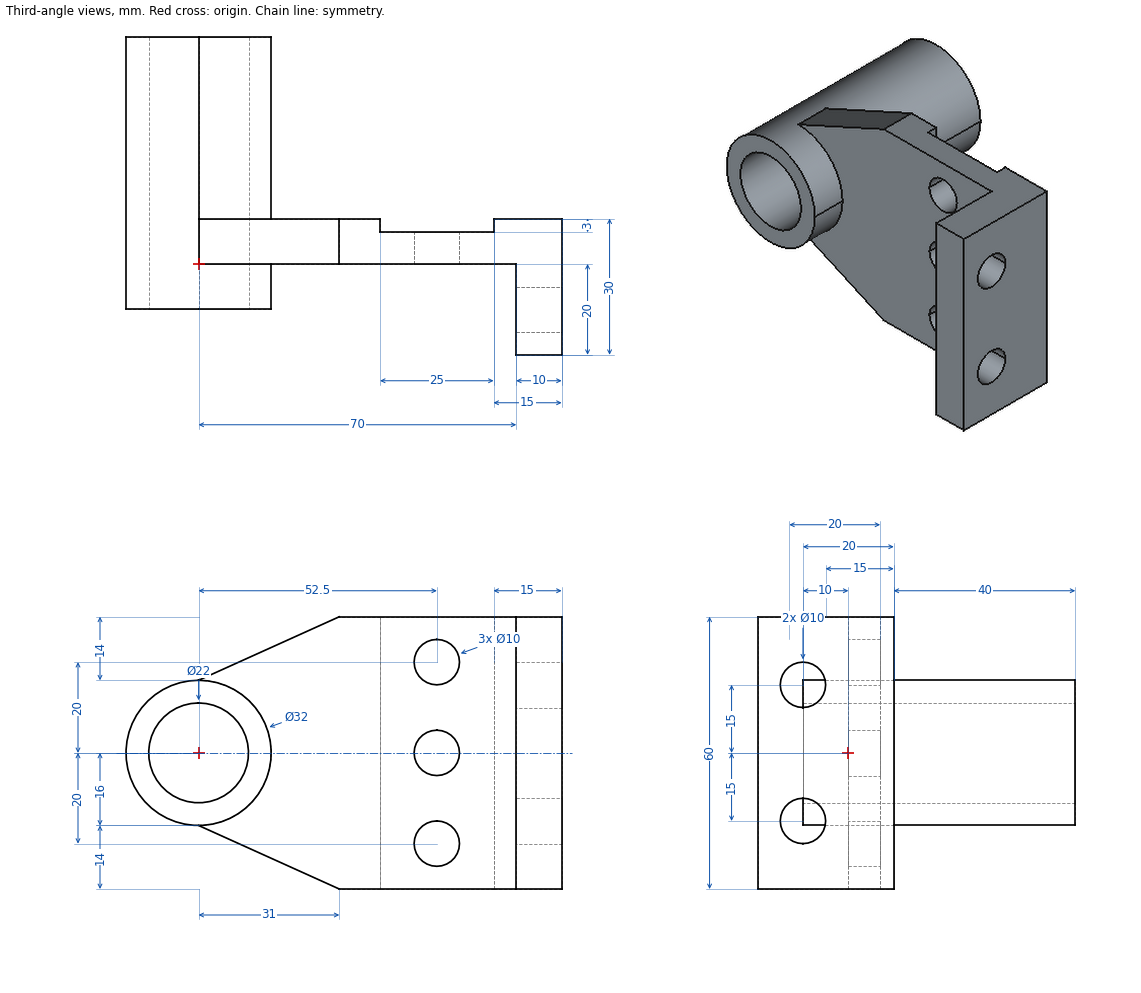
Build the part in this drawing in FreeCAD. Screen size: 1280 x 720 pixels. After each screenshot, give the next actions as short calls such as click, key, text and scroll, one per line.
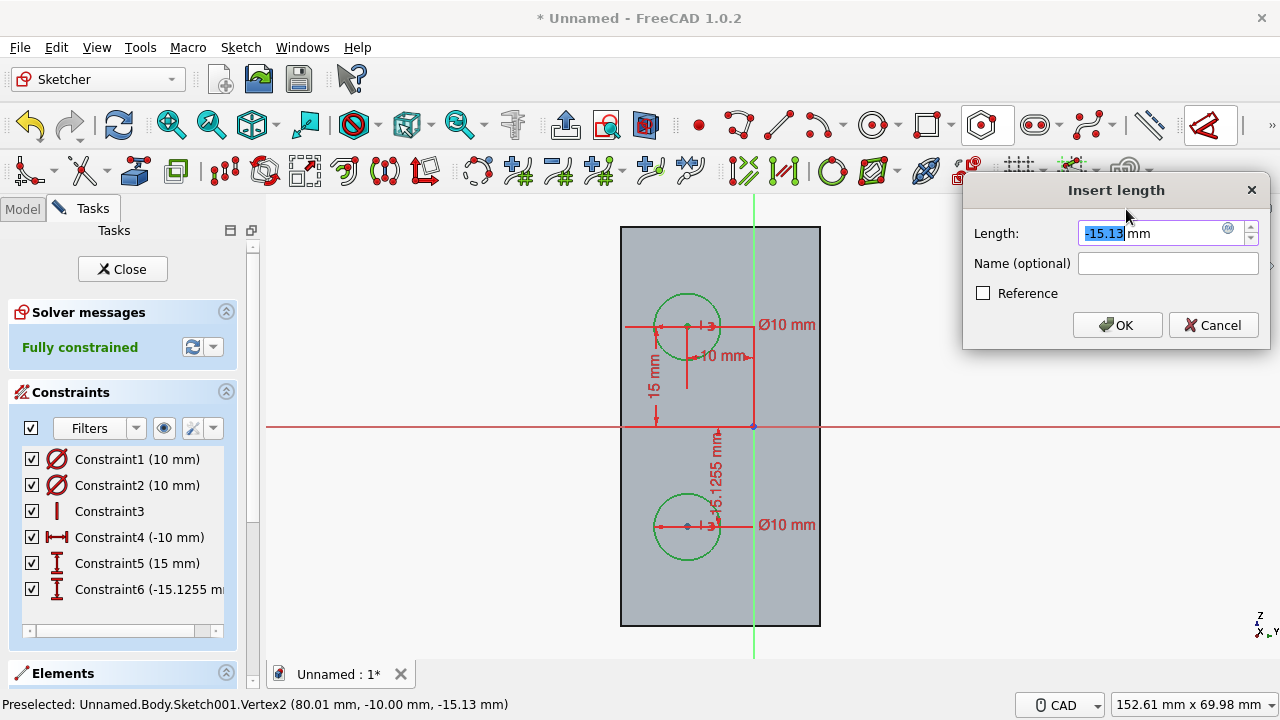
text(-15)
key(Return)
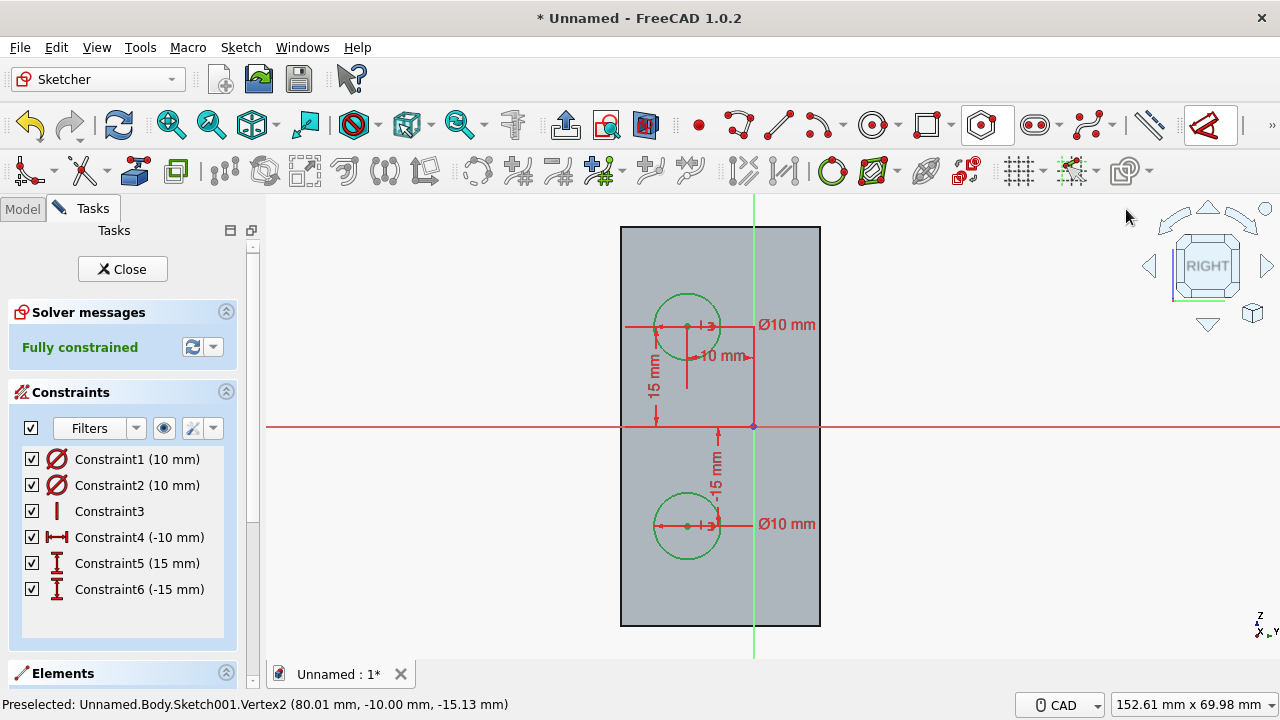
click(123, 269)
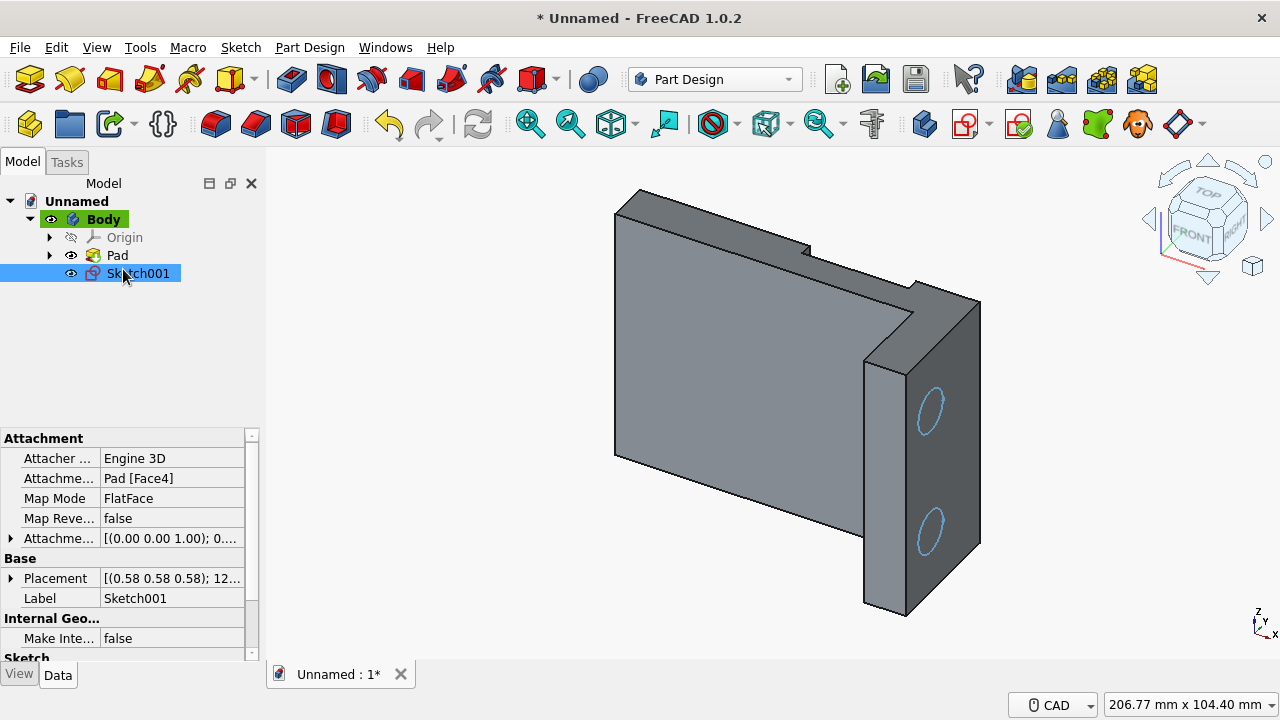
click(292, 80)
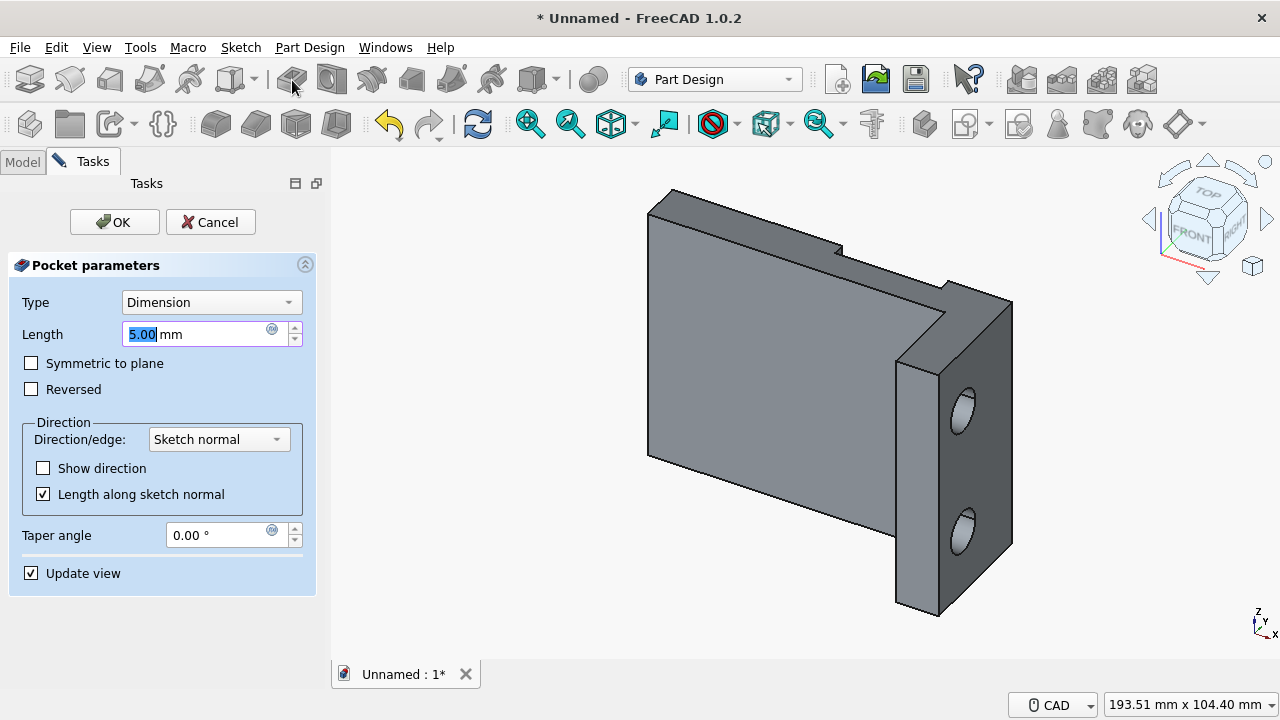
text(15)
key(Tab)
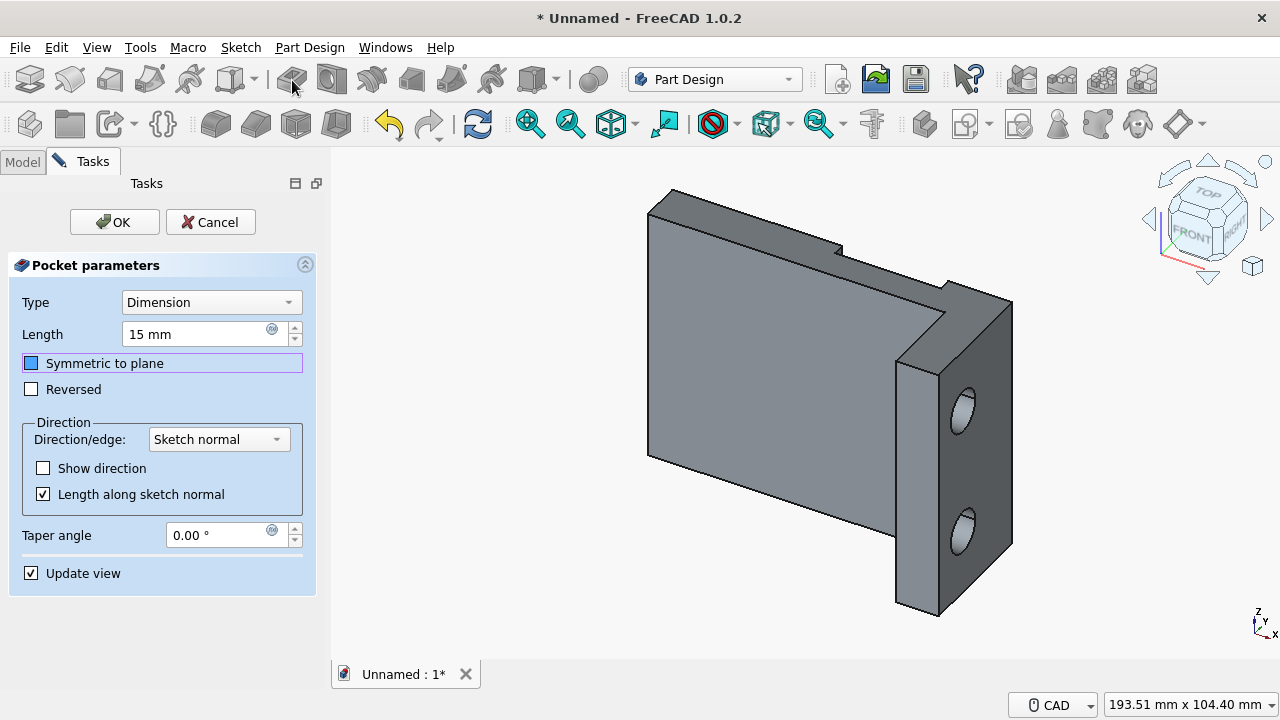
click(115, 222)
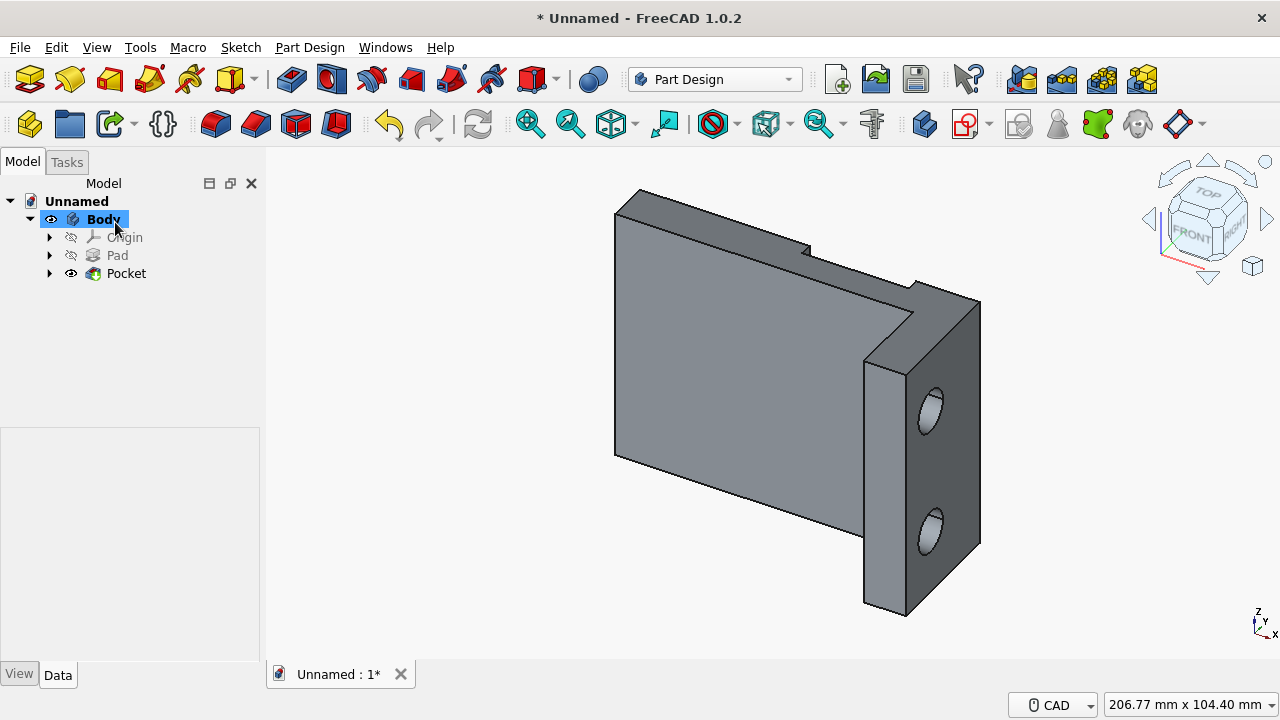
key(4)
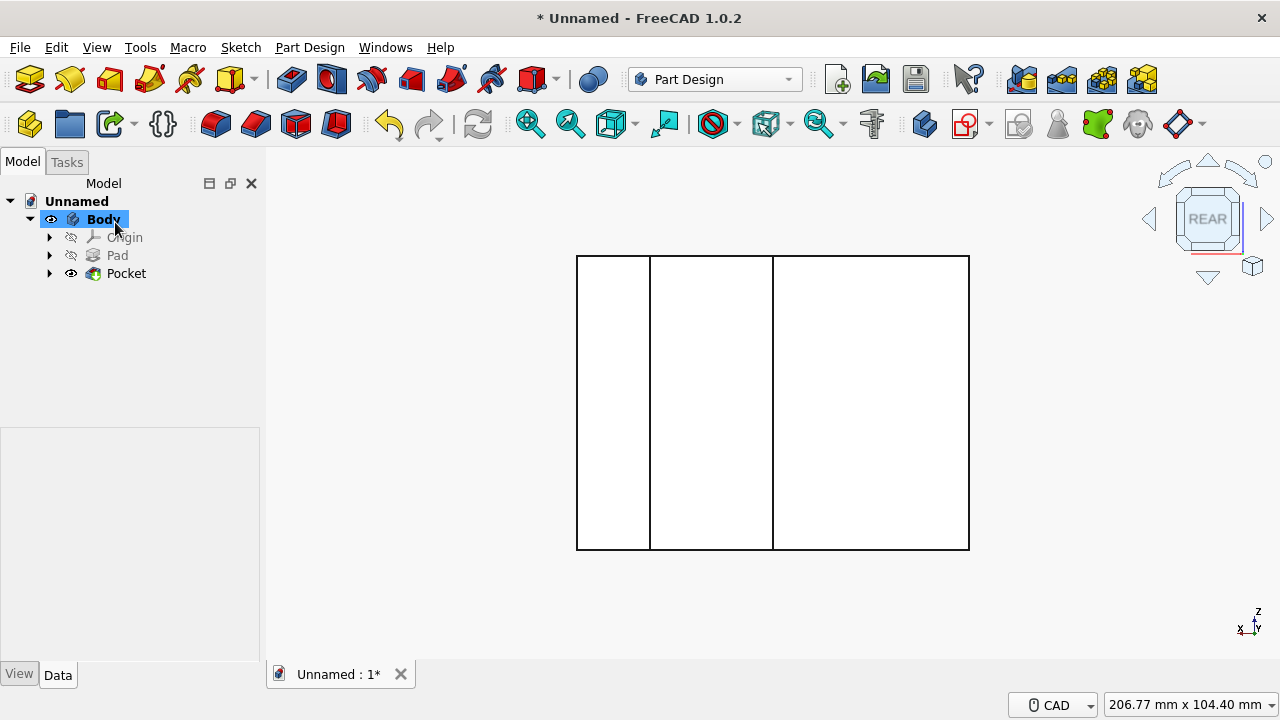
click(871, 360)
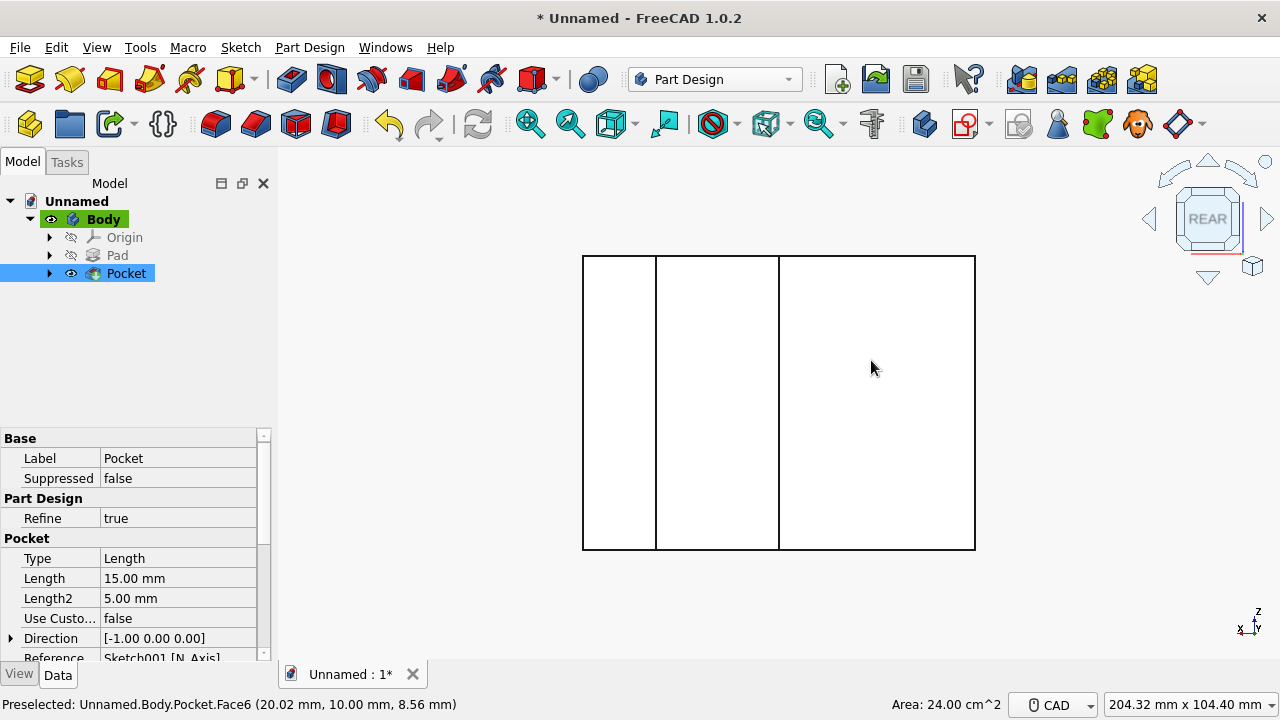
click(966, 124)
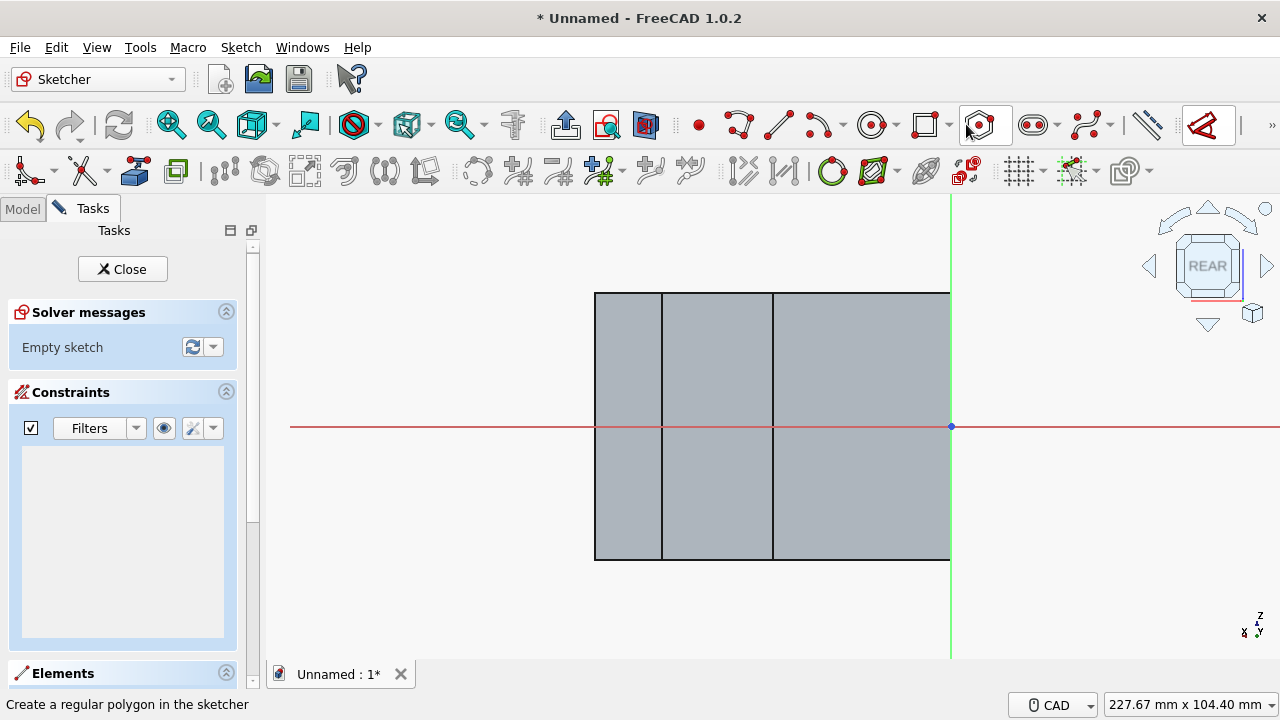
click(740, 126)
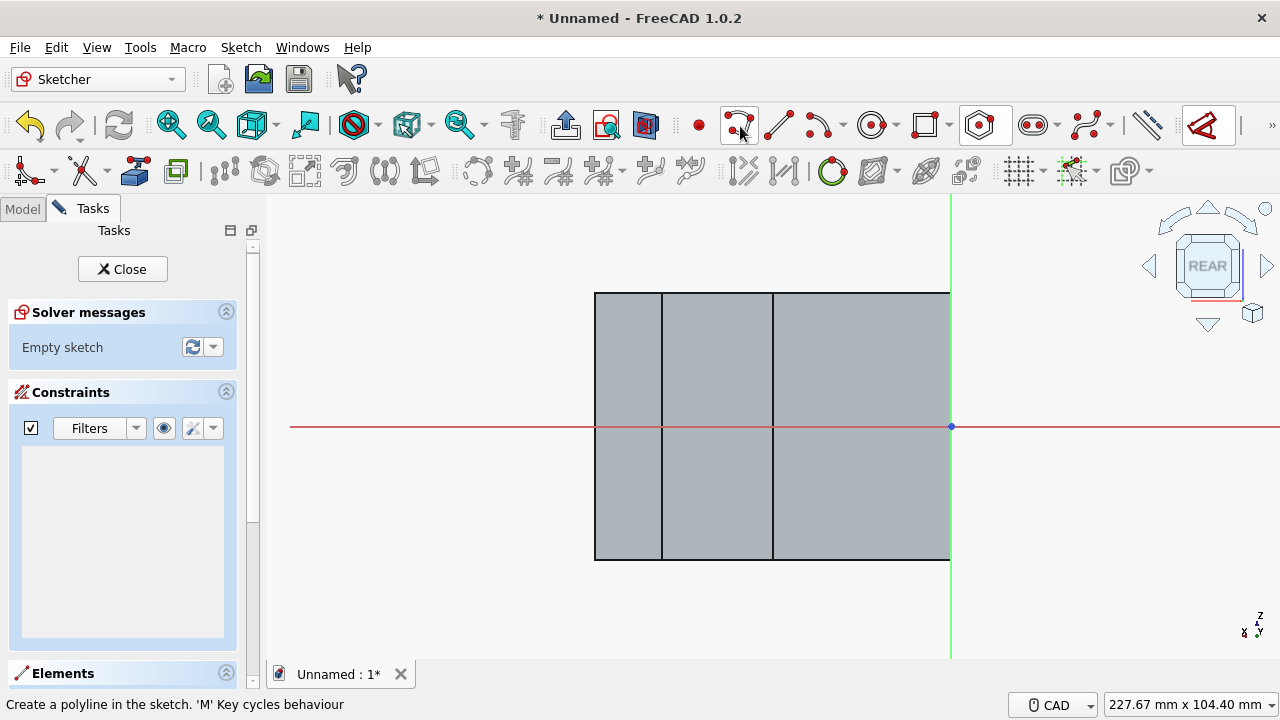
click(951, 498)
click(813, 560)
click(942, 560)
click(951, 499)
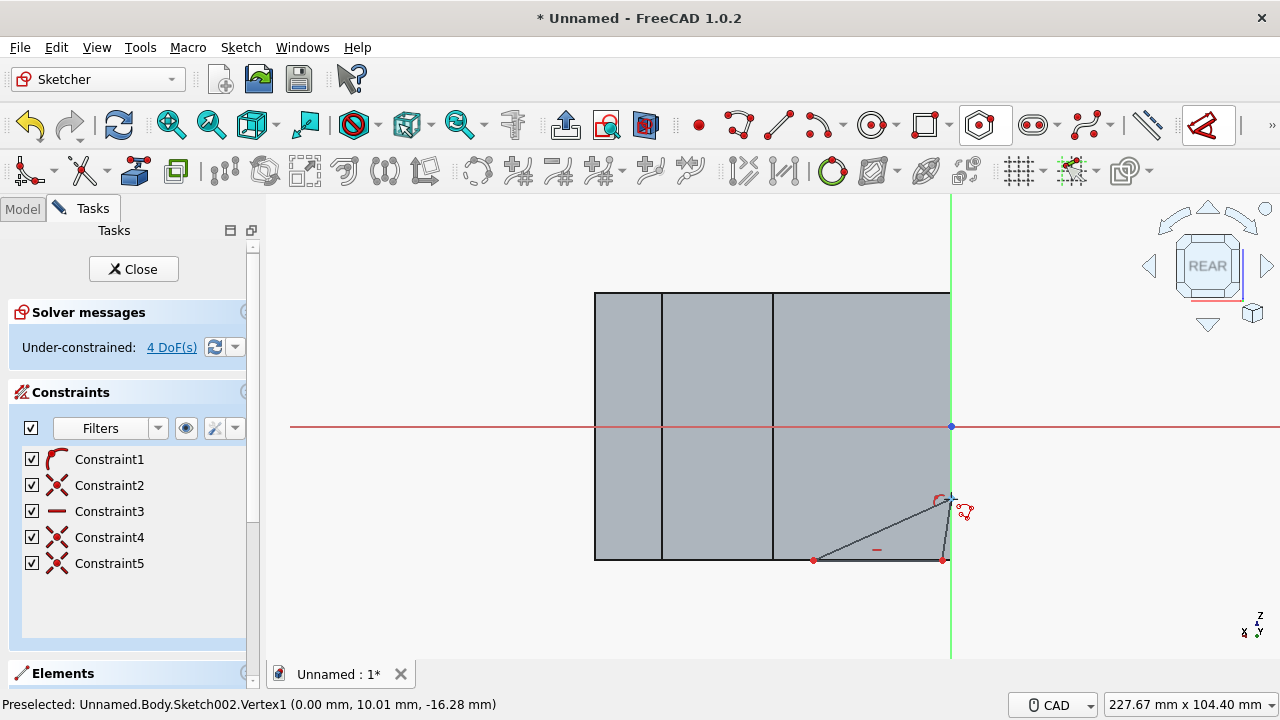
click(951, 355)
click(942, 293)
click(813, 293)
click(951, 356)
key(Escape)
key(Escape)